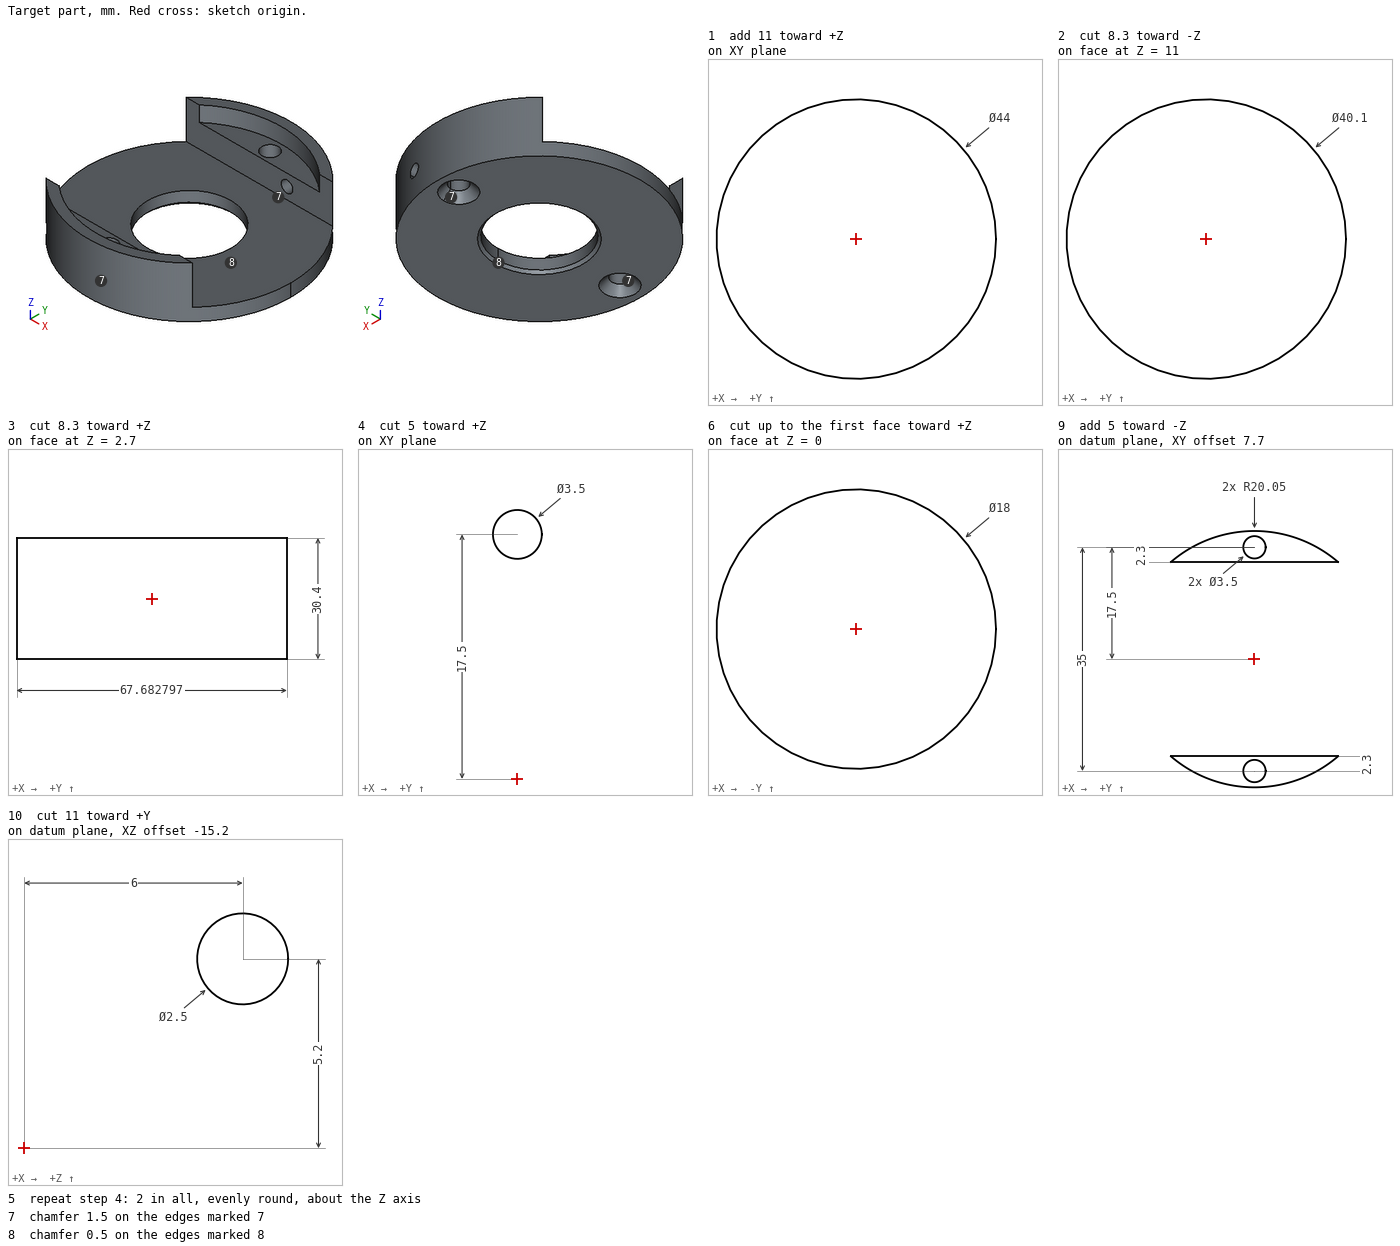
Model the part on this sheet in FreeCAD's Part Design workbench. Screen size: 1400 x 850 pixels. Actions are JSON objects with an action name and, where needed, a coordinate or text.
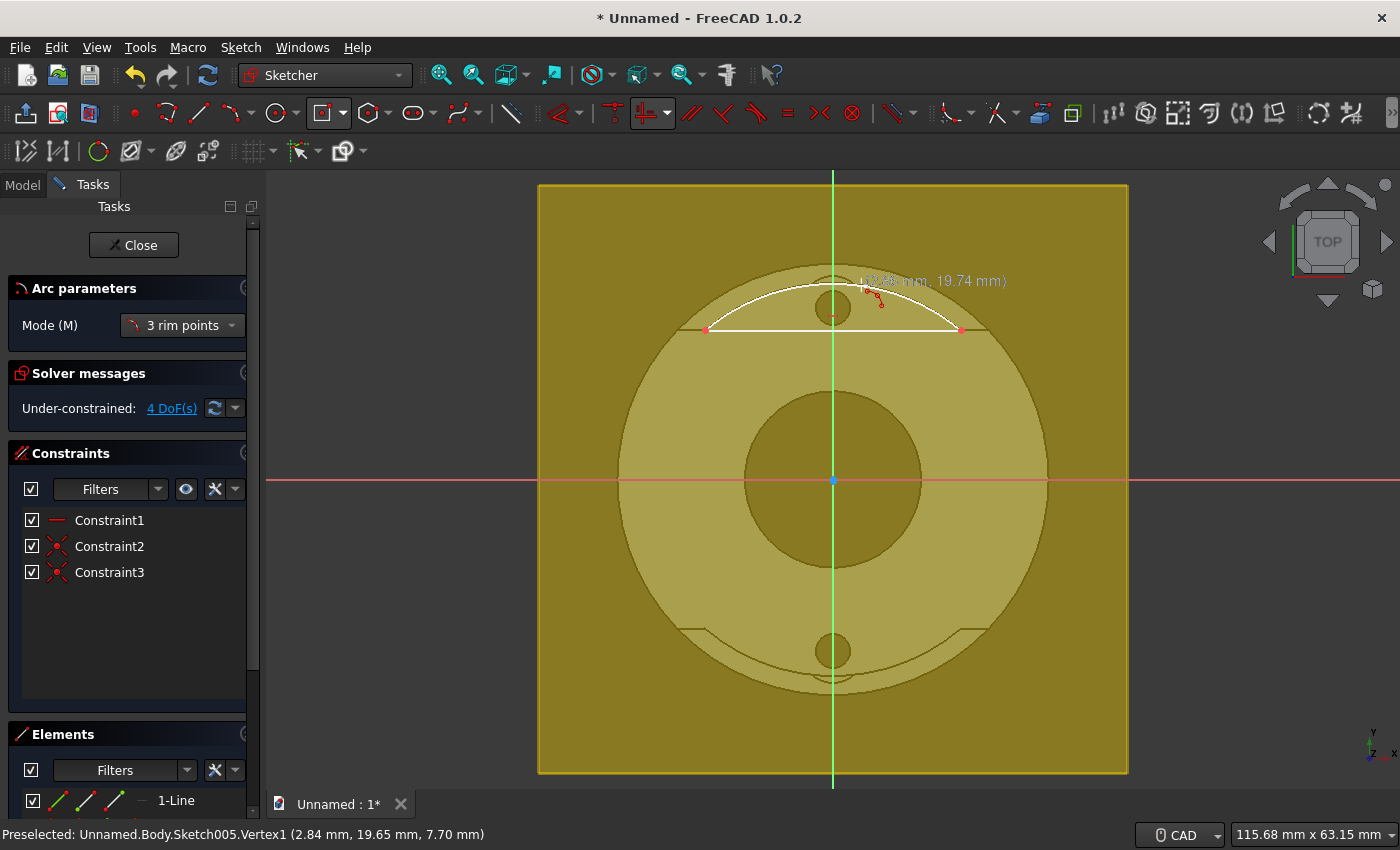
{"action": "key", "text": "g l"}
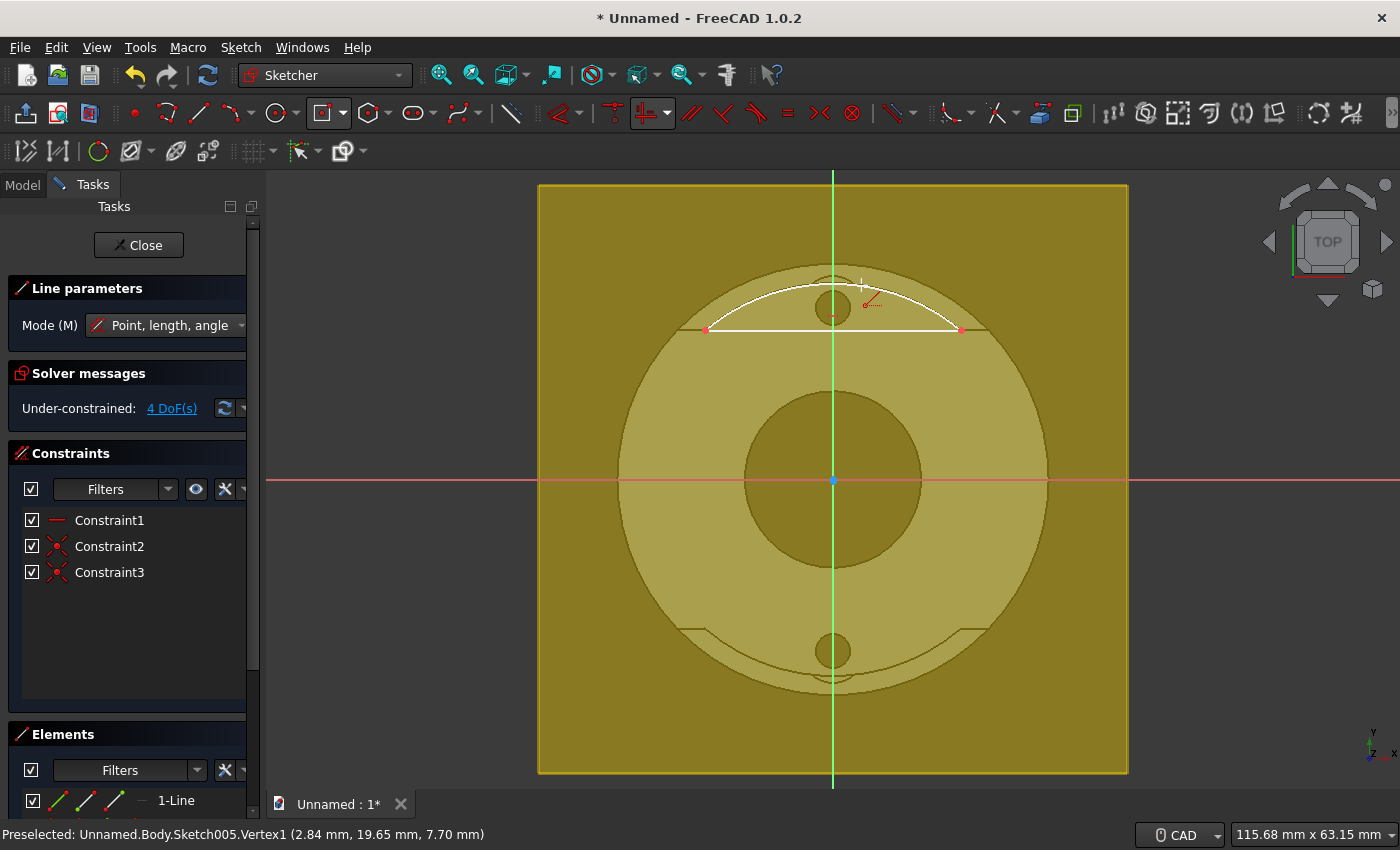
{"action": "left_click", "coordinate": [961, 629]}
{"action": "left_click", "coordinate": [705, 629]}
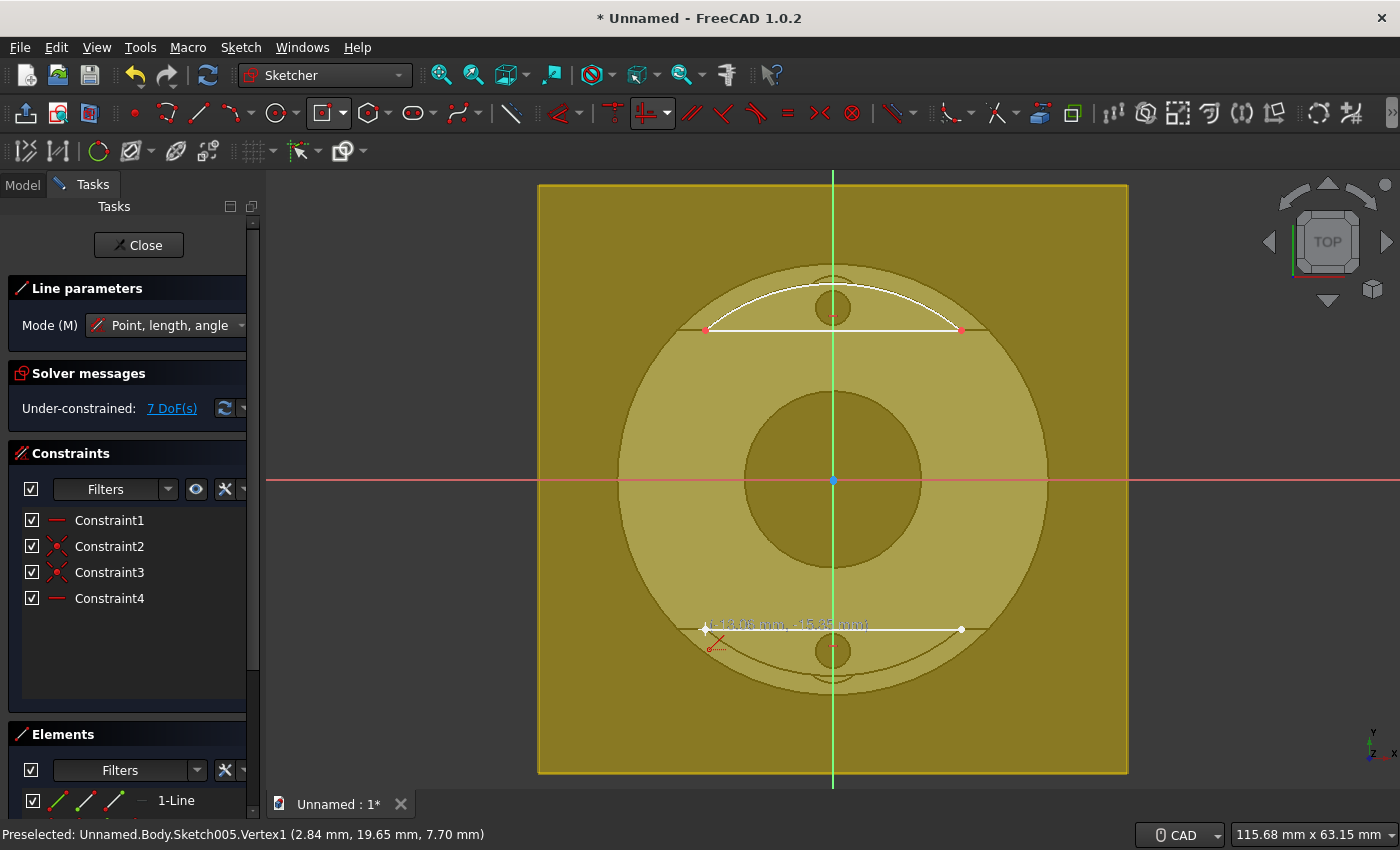
{"action": "key", "text": "g 3 a"}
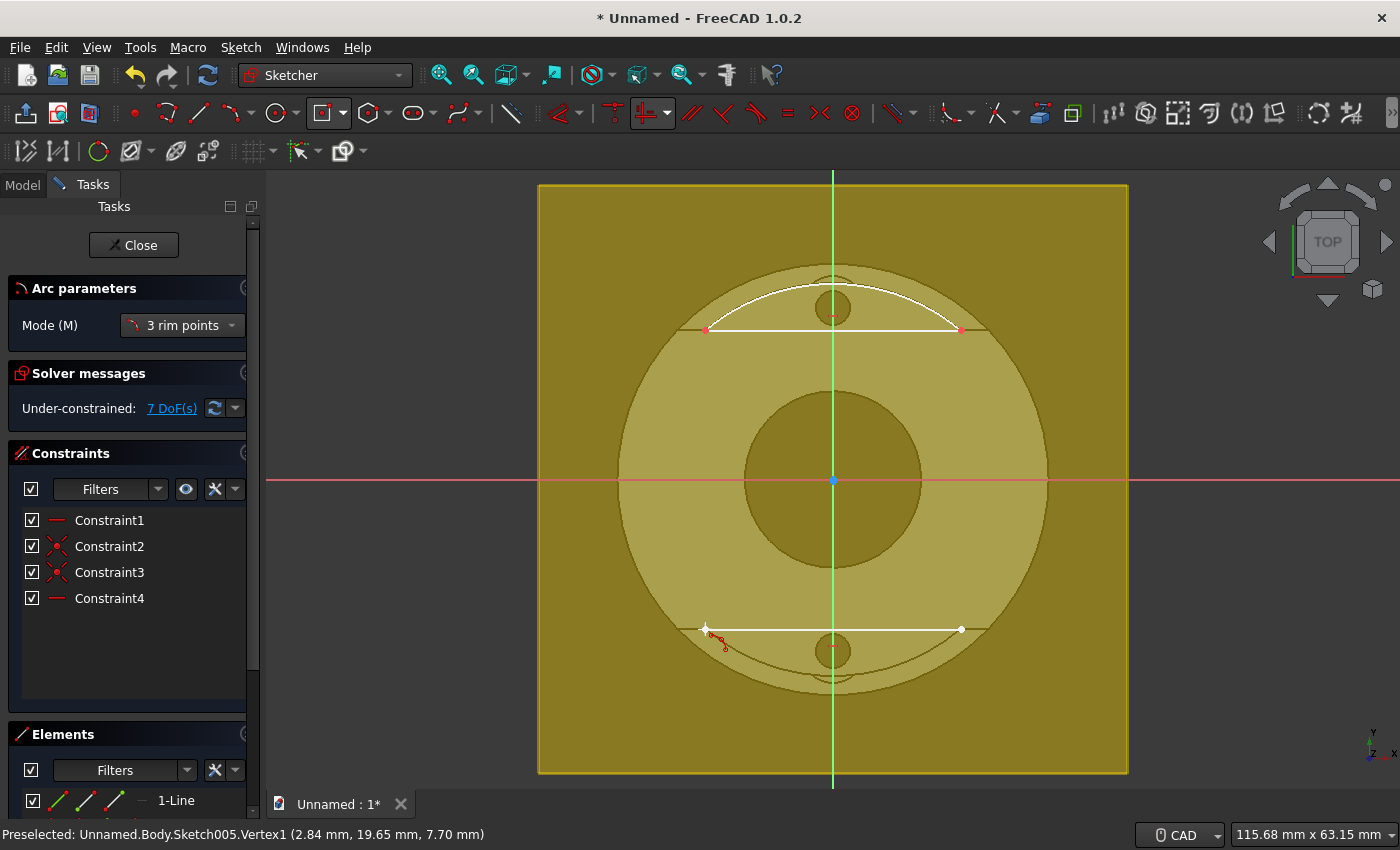
{"action": "left_click", "coordinate": [705, 630]}
{"action": "left_click", "coordinate": [961, 630]}
{"action": "left_click", "coordinate": [805, 674]}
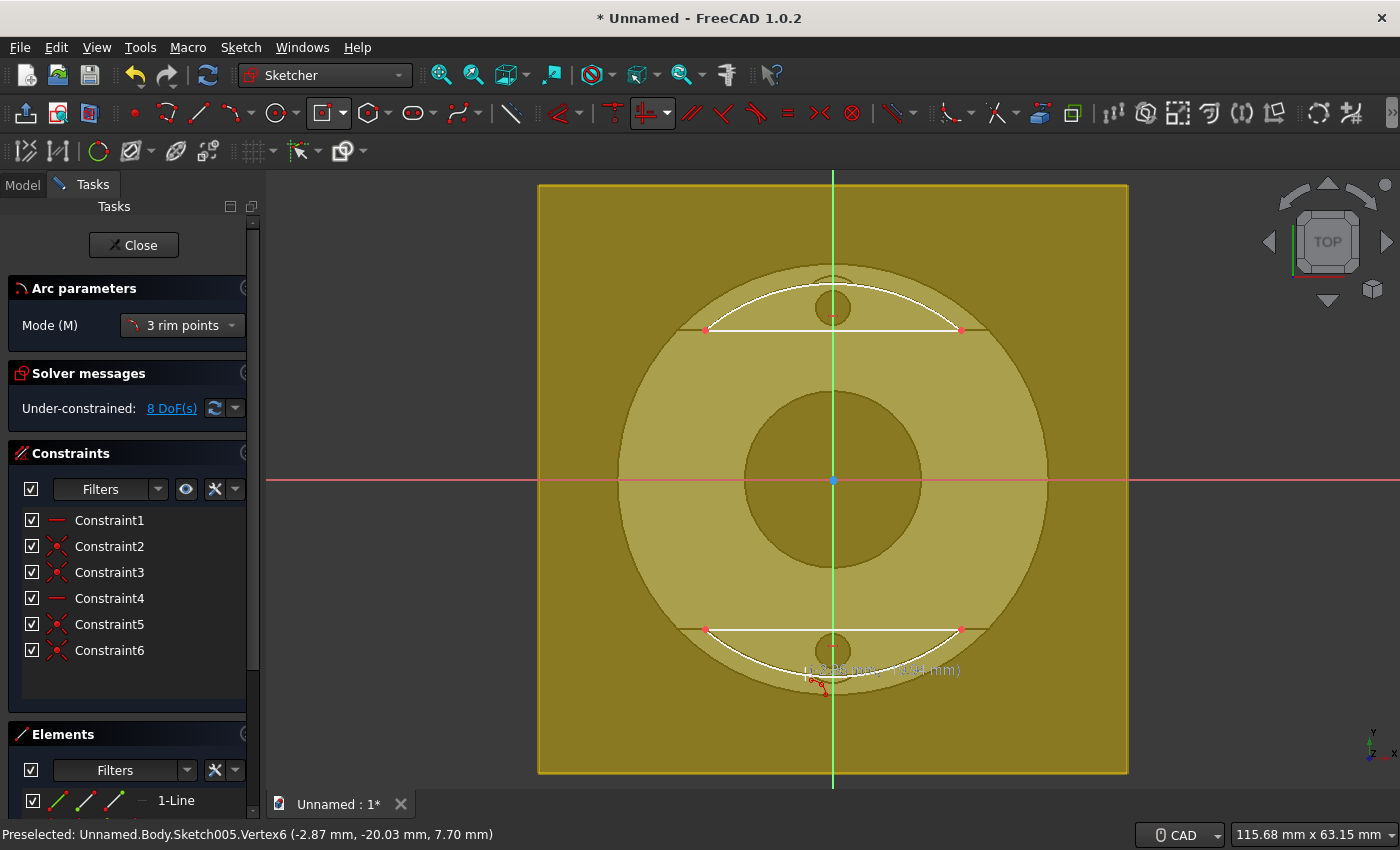
{"action": "key", "text": "g c"}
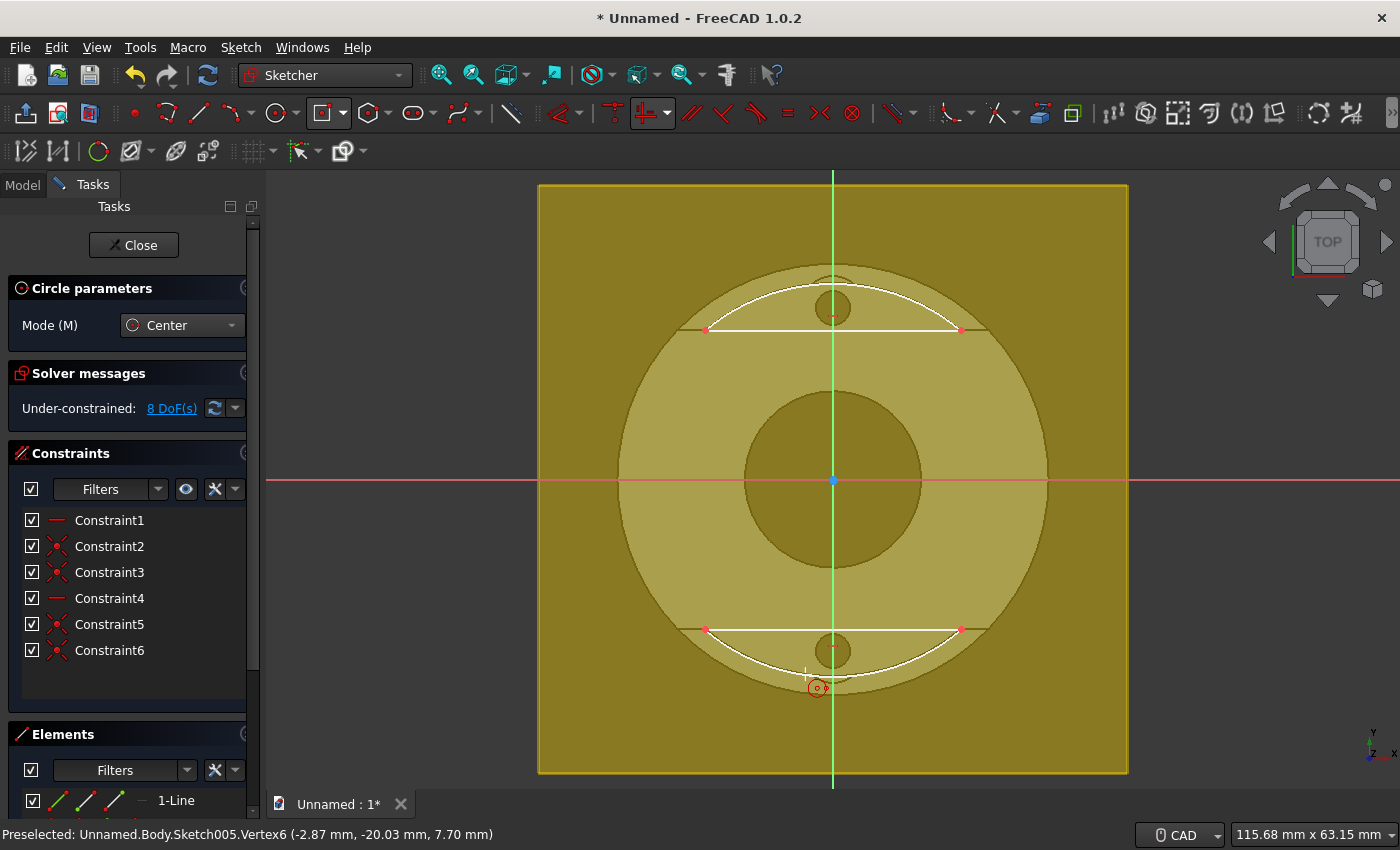
{"action": "scroll", "coordinate": [833, 308], "scroll_direction": "up", "scroll_amount": 2}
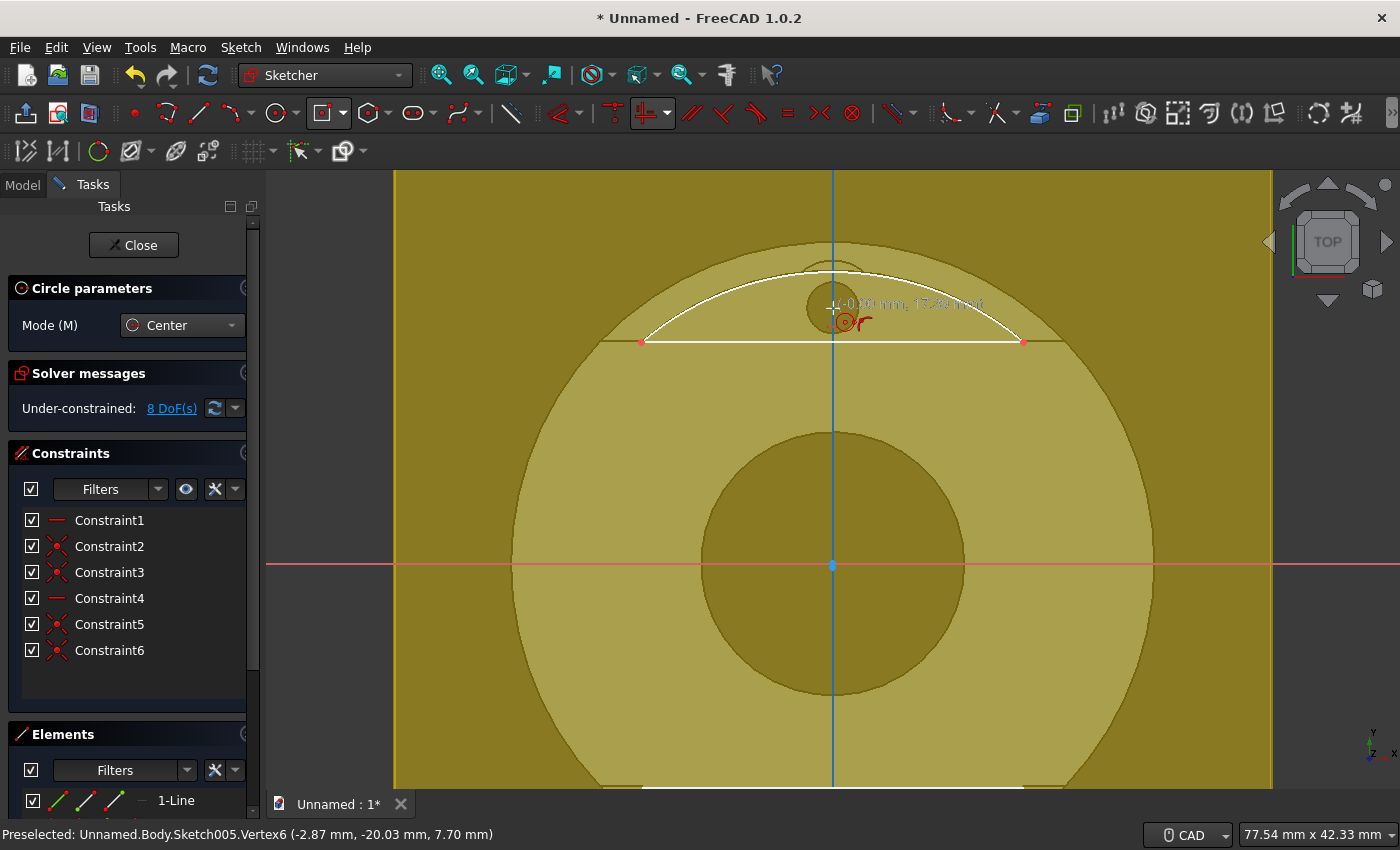
{"action": "left_click", "coordinate": [833, 308]}
{"action": "left_click", "coordinate": [851, 290]}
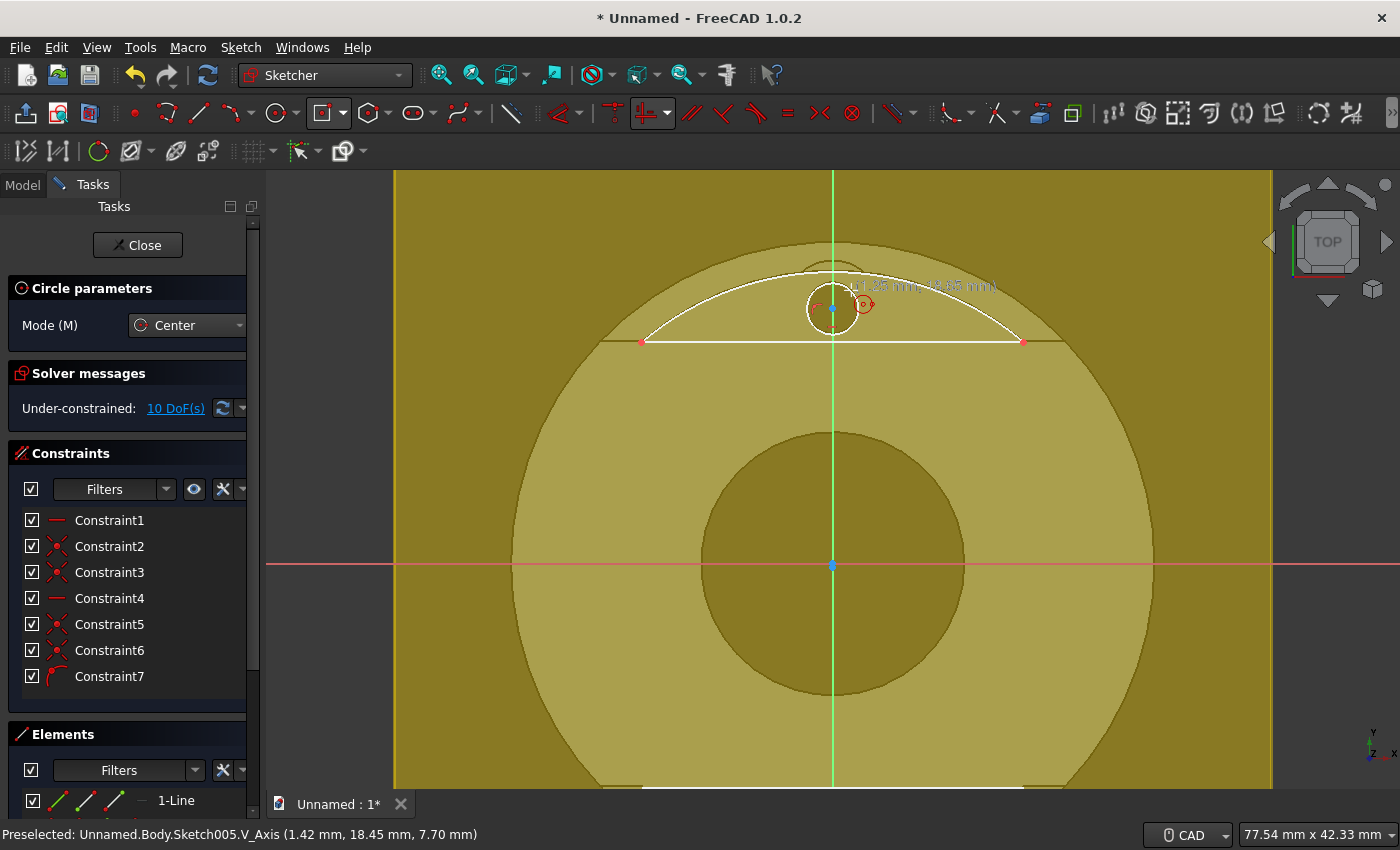
{"action": "scroll", "coordinate": [626, 308], "scroll_direction": "down", "scroll_amount": 2}